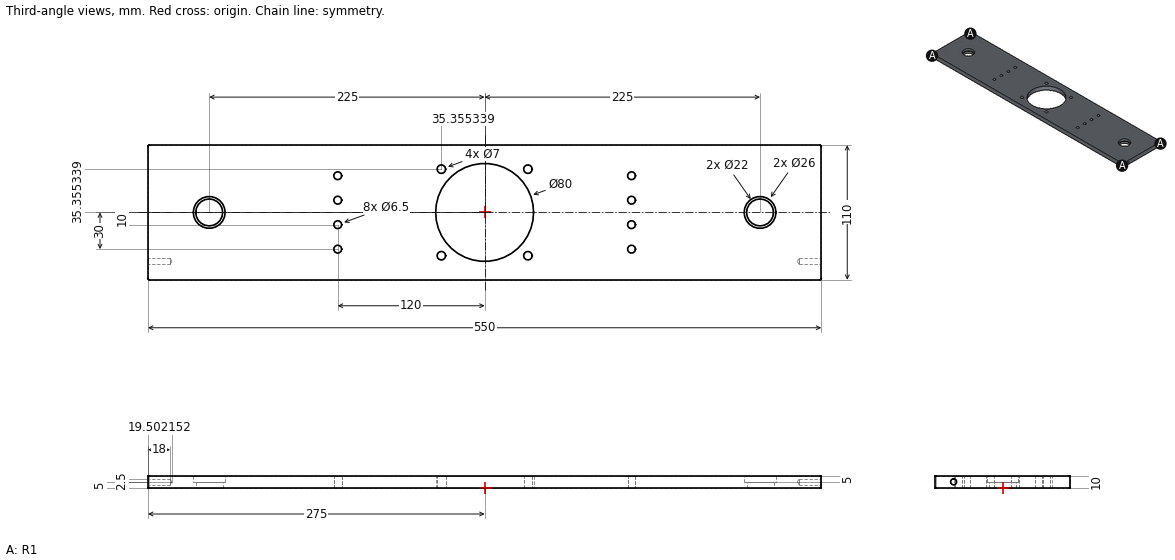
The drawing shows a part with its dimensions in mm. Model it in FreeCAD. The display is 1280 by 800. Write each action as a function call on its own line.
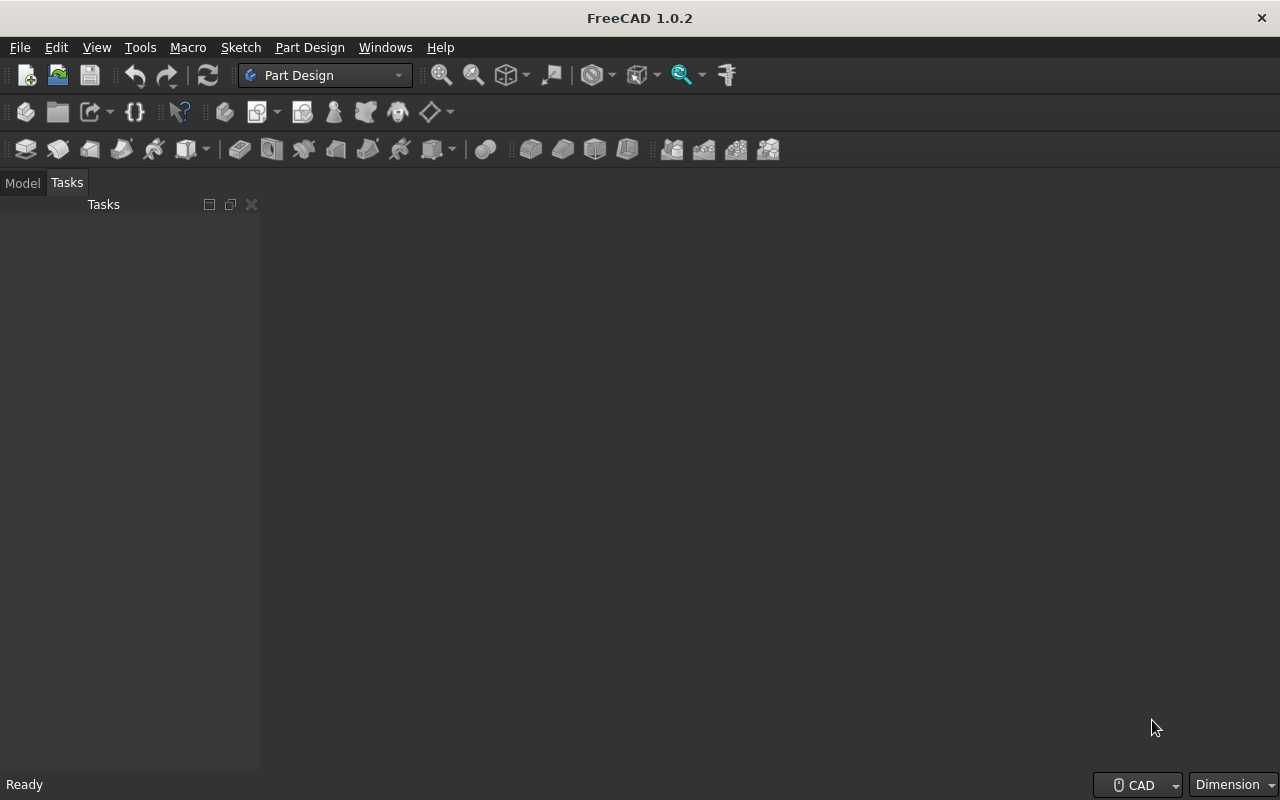
click(26, 76)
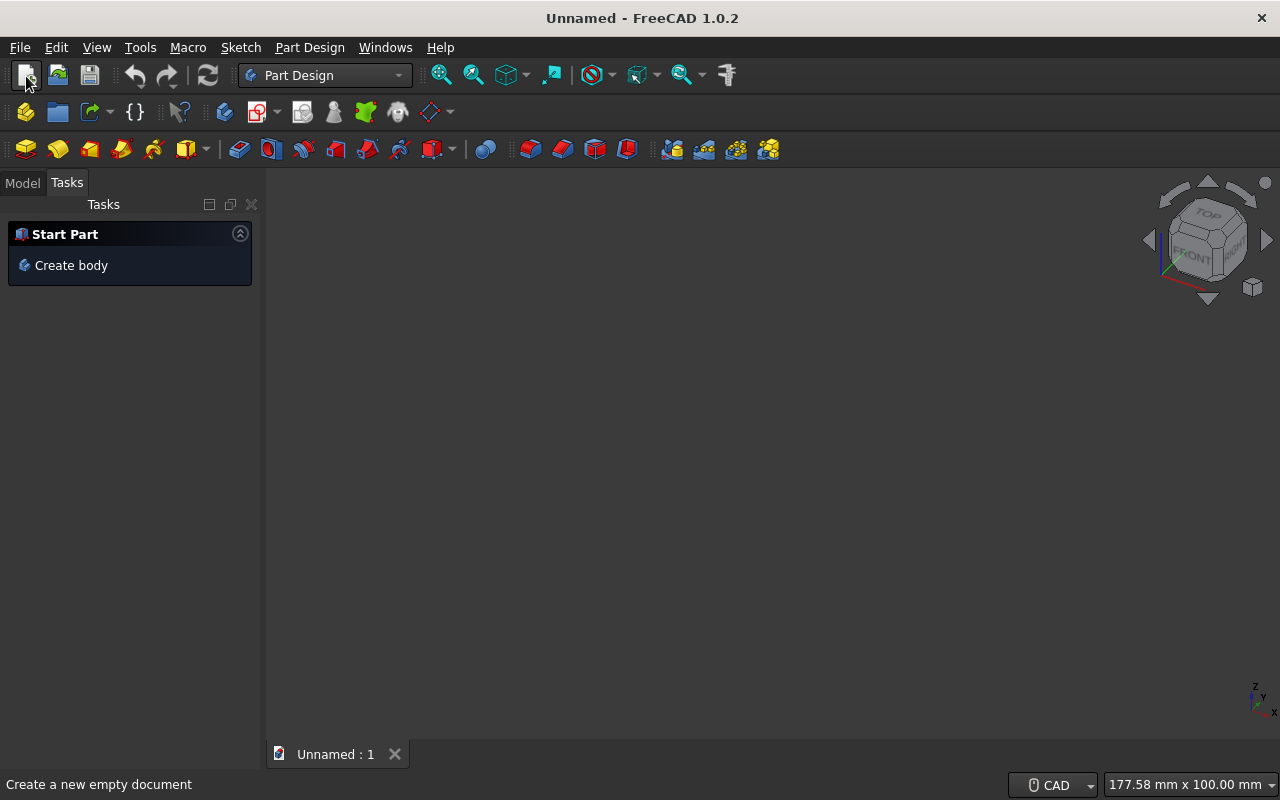
click(258, 112)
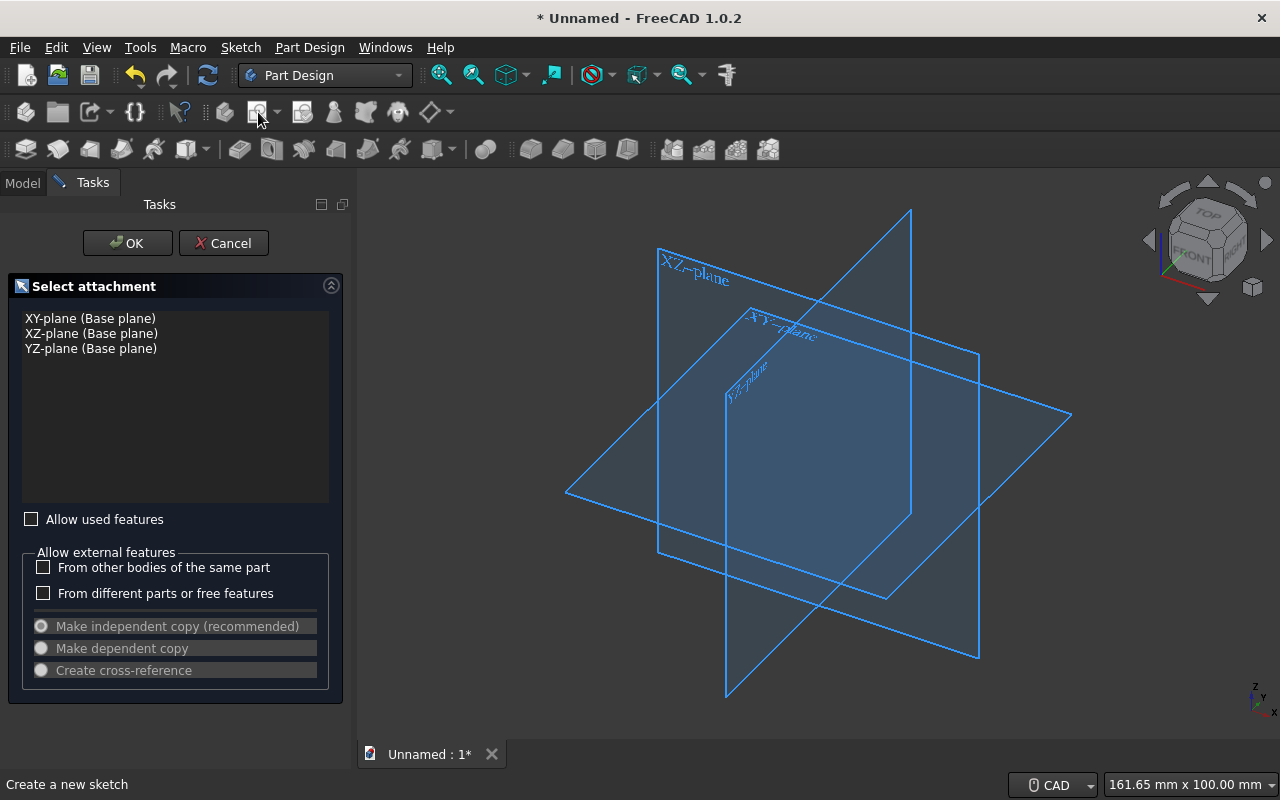
click(82, 318)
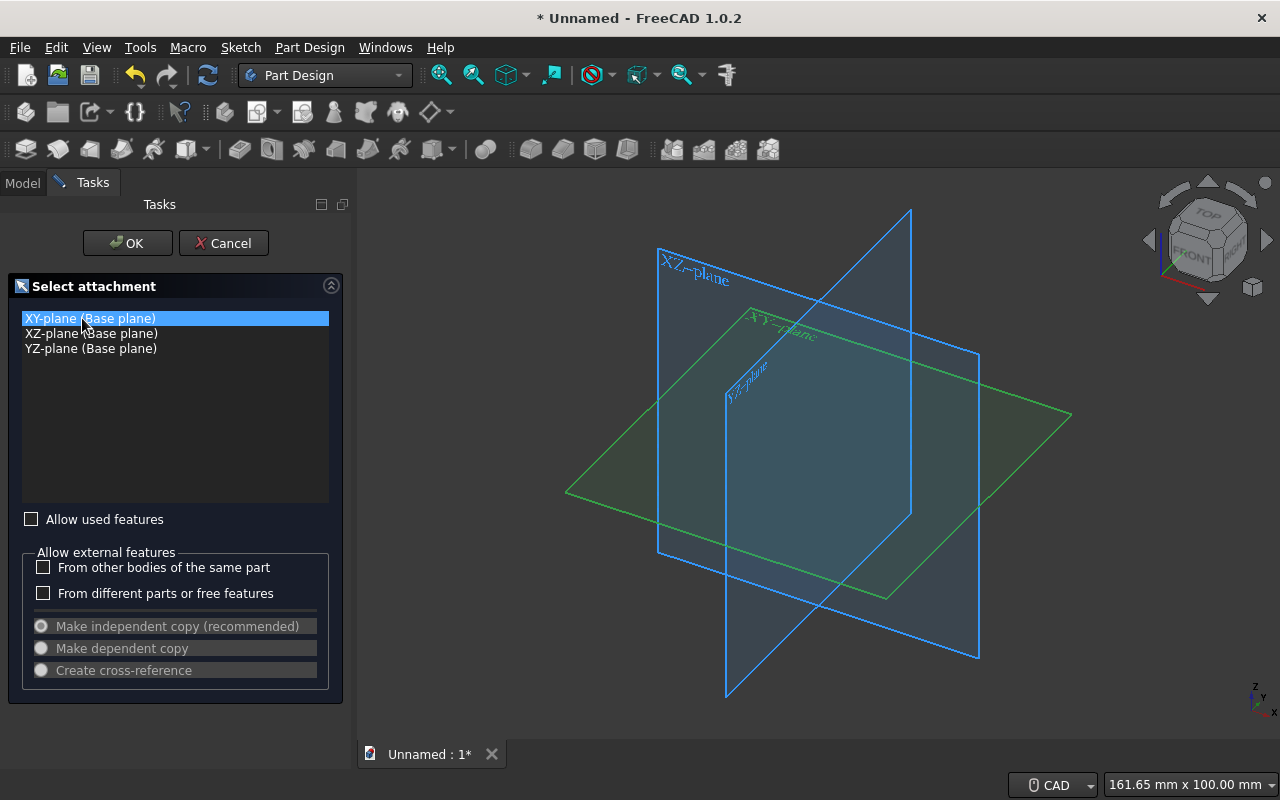
click(128, 243)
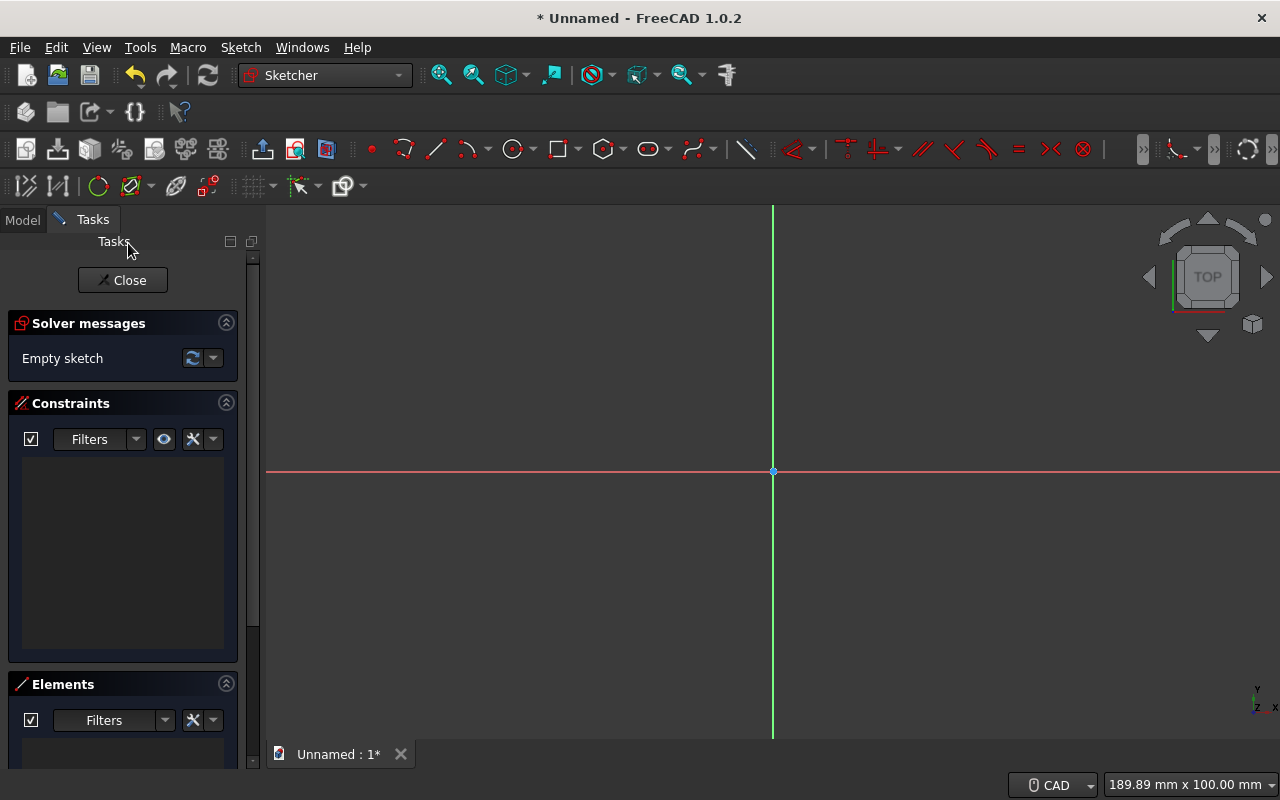
scroll(687, 472, down, 8)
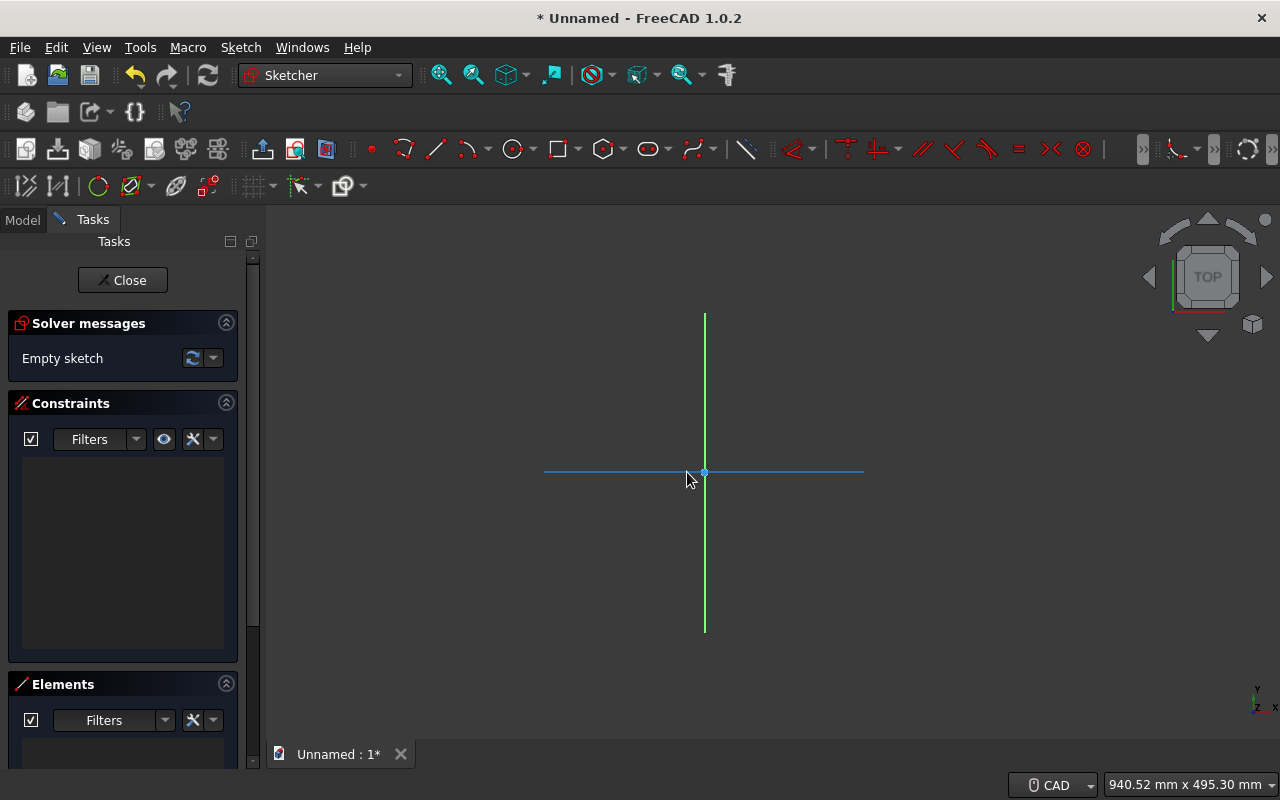
key(g)
key(v)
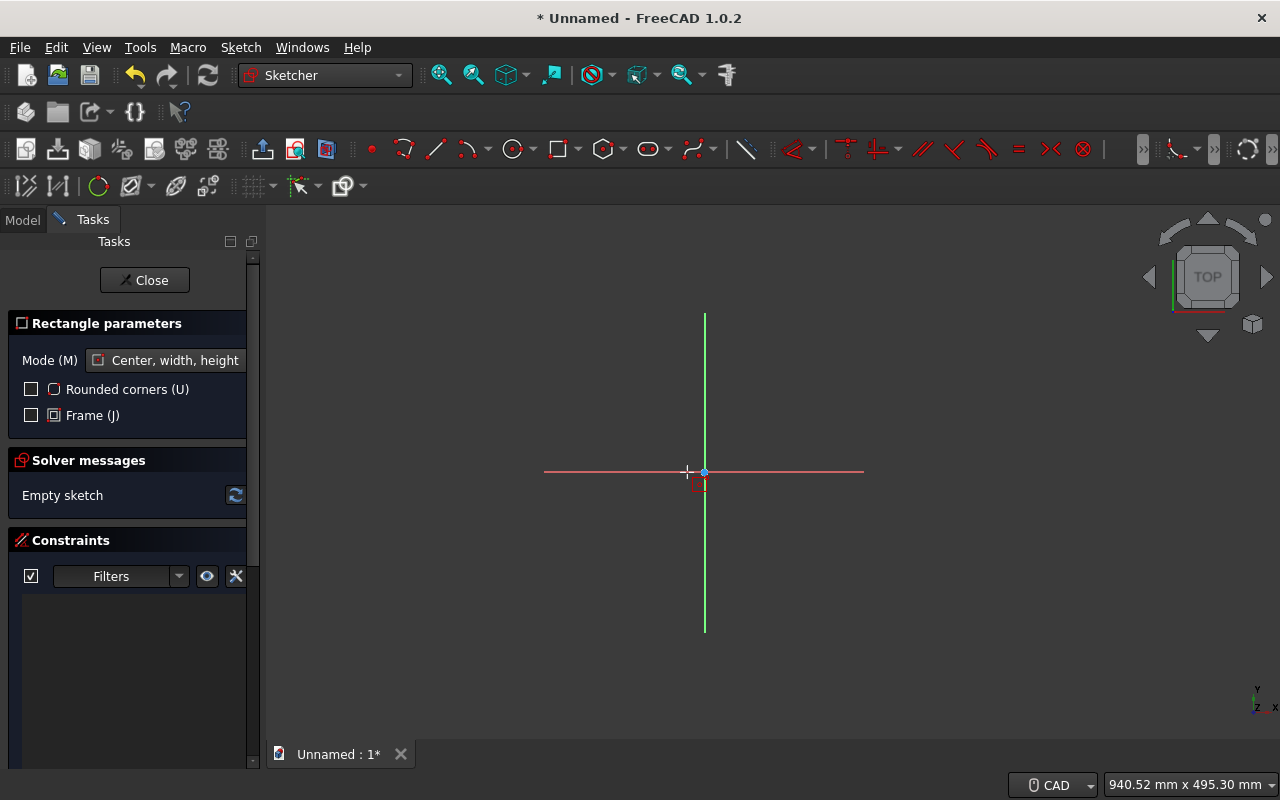
click(705, 472)
move(1001, 413)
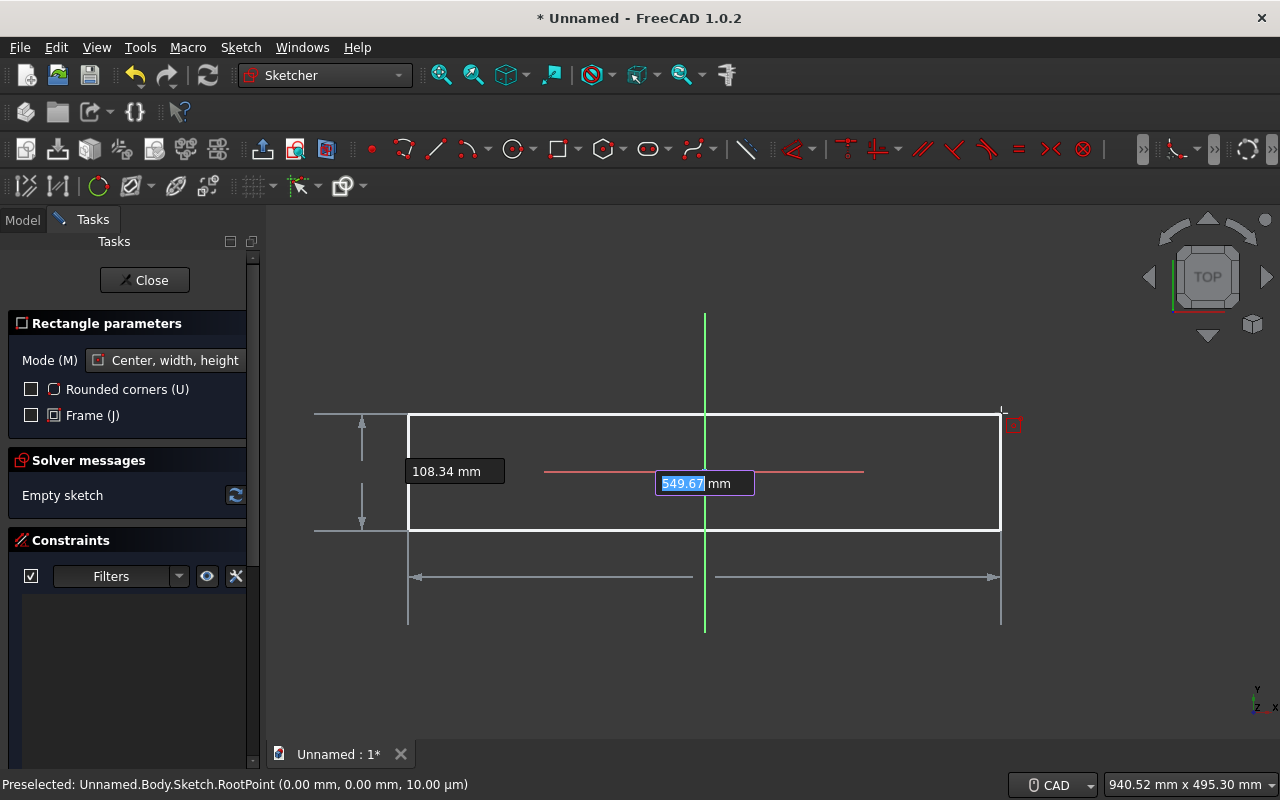
text(550)
key(Tab)
text(110)
key(Return)
key(Escape)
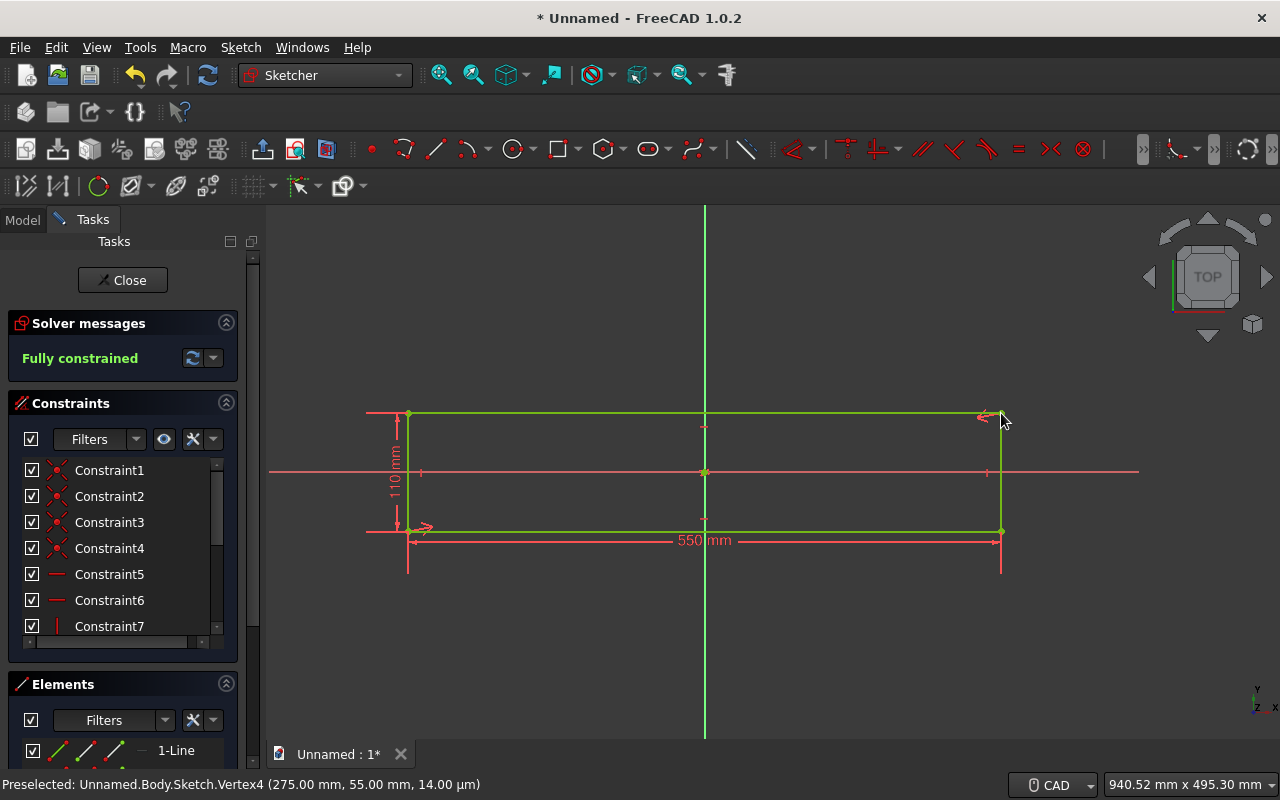
click(123, 280)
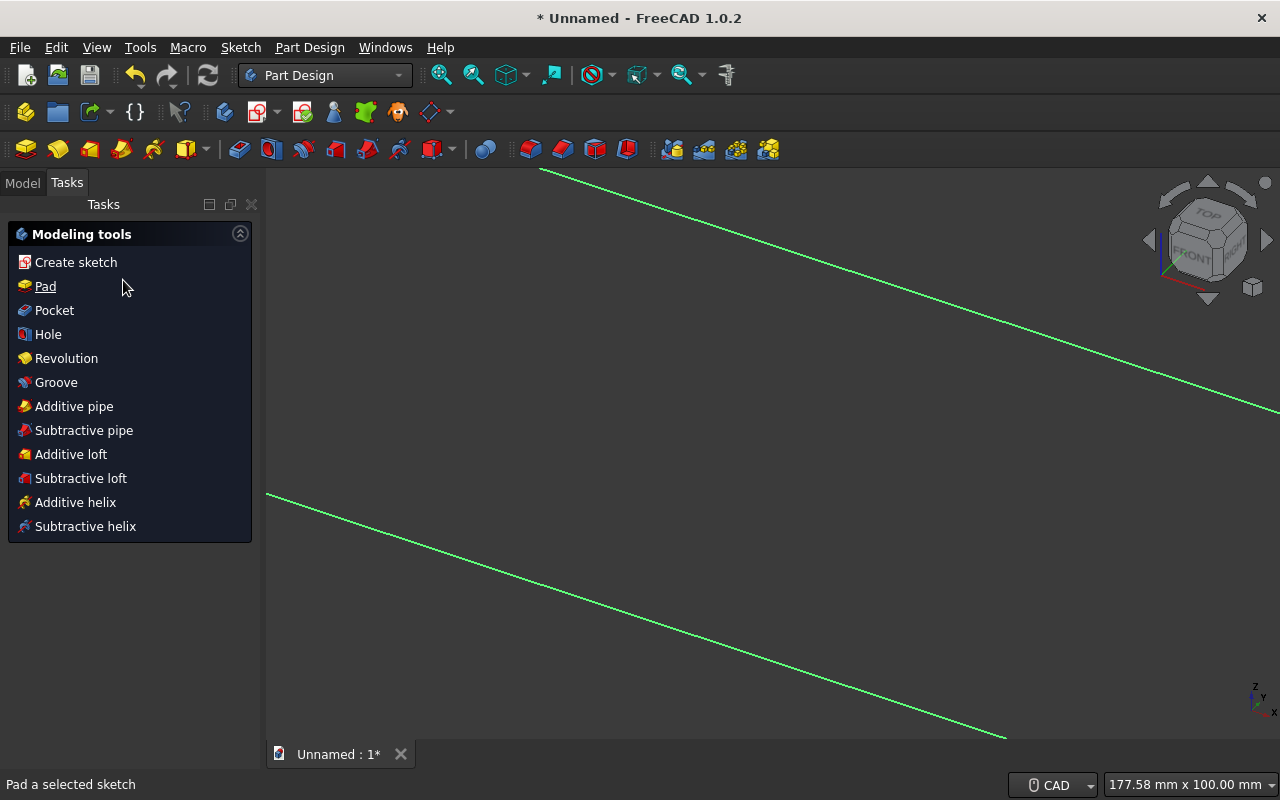
click(26, 150)